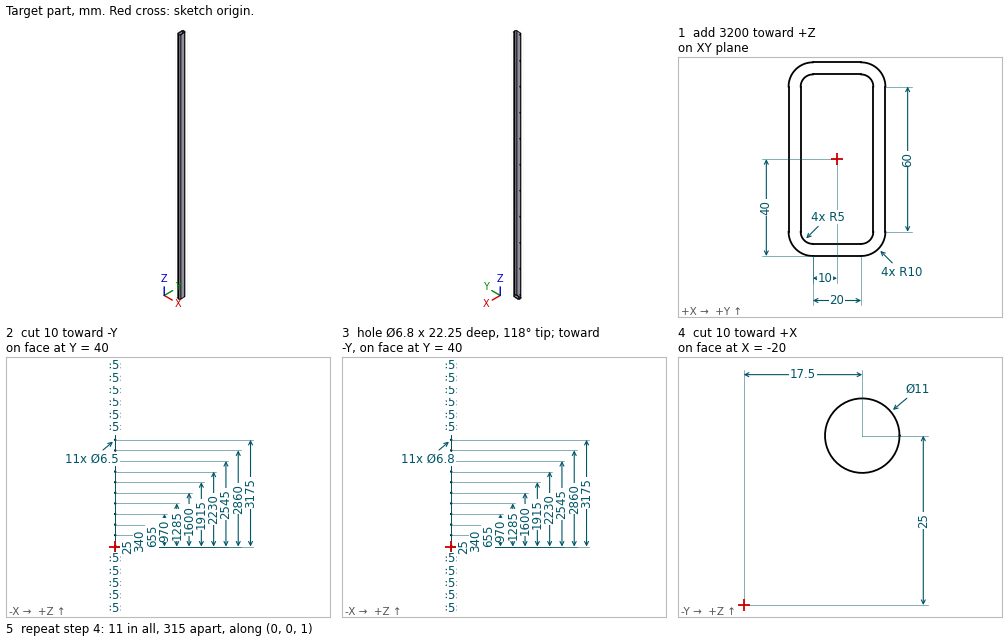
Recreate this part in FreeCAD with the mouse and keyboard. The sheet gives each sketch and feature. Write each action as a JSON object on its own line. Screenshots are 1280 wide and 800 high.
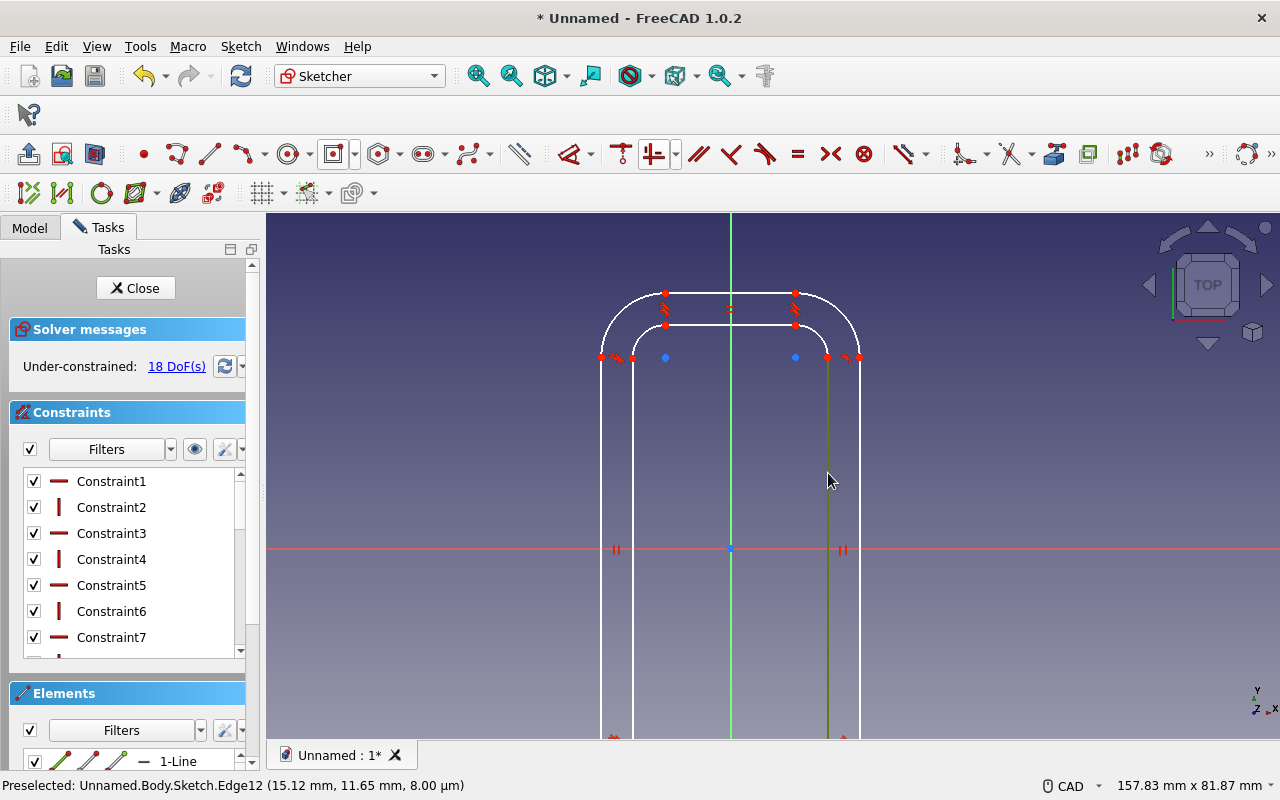
{"action": "left_click", "coordinate": [824, 343]}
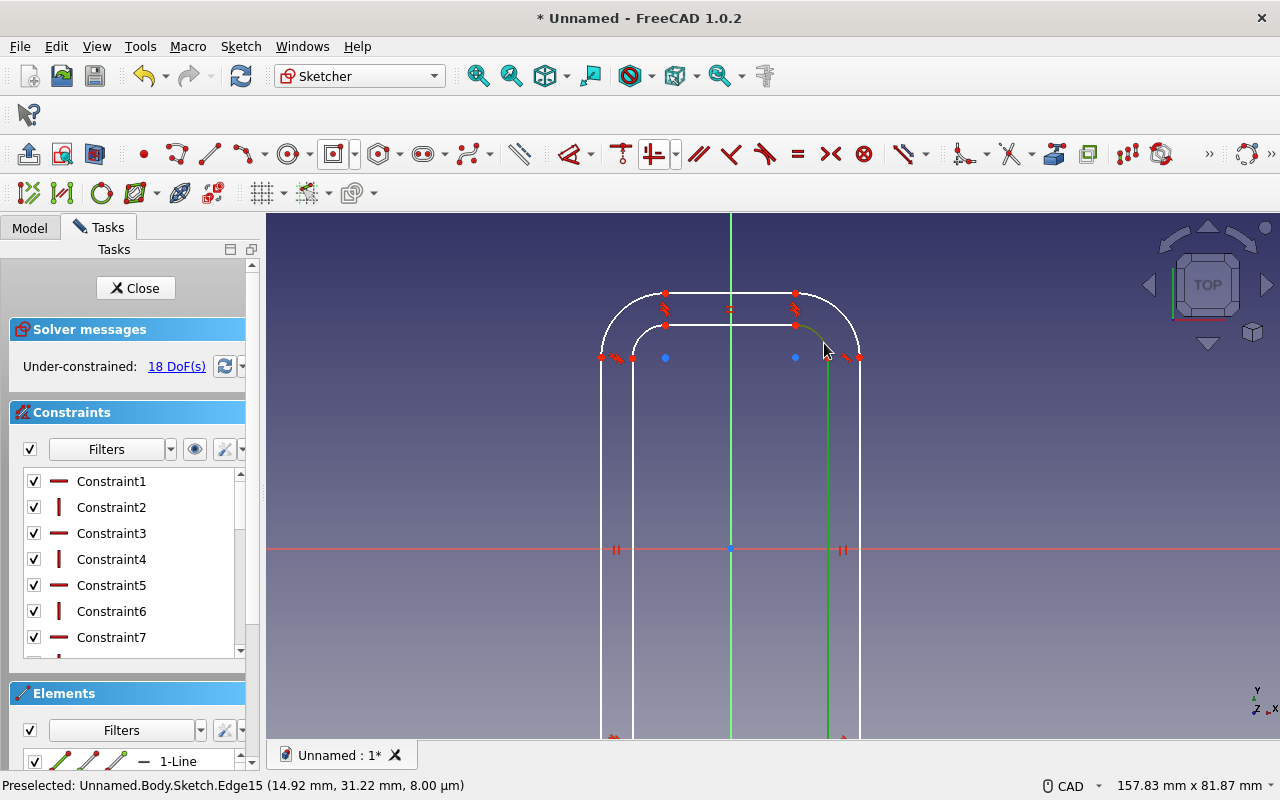
{"action": "left_click", "coordinate": [765, 154]}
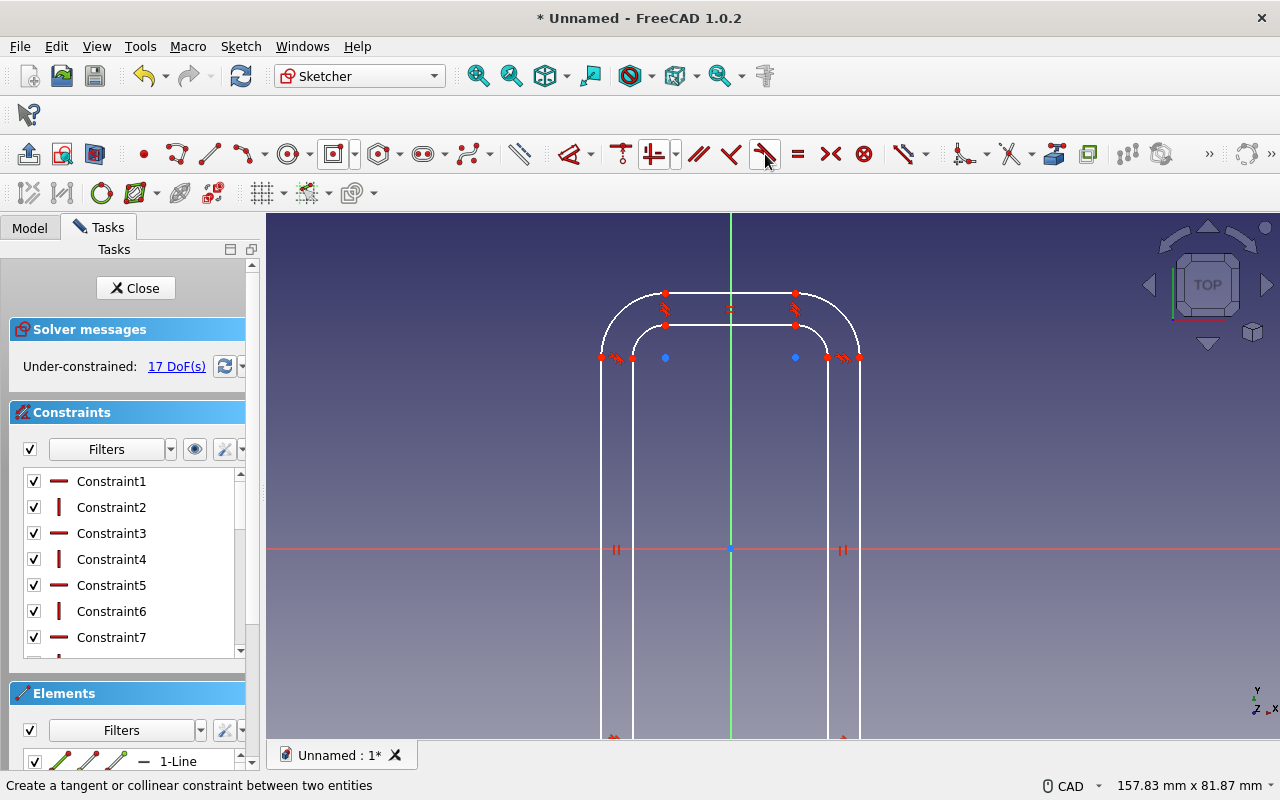
{"action": "left_click", "coordinate": [828, 473]}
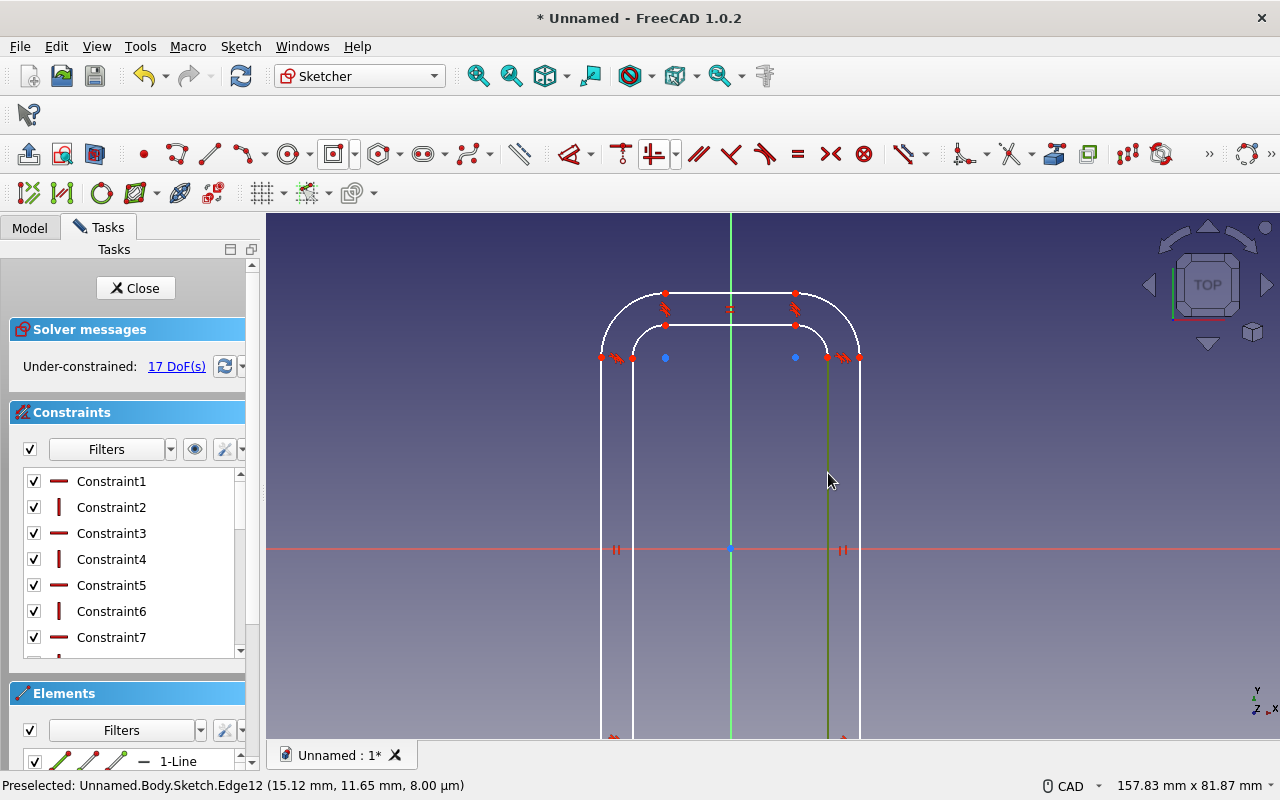
{"action": "scroll", "coordinate": [651, 328], "scroll_direction": "down", "scroll_amount": 2}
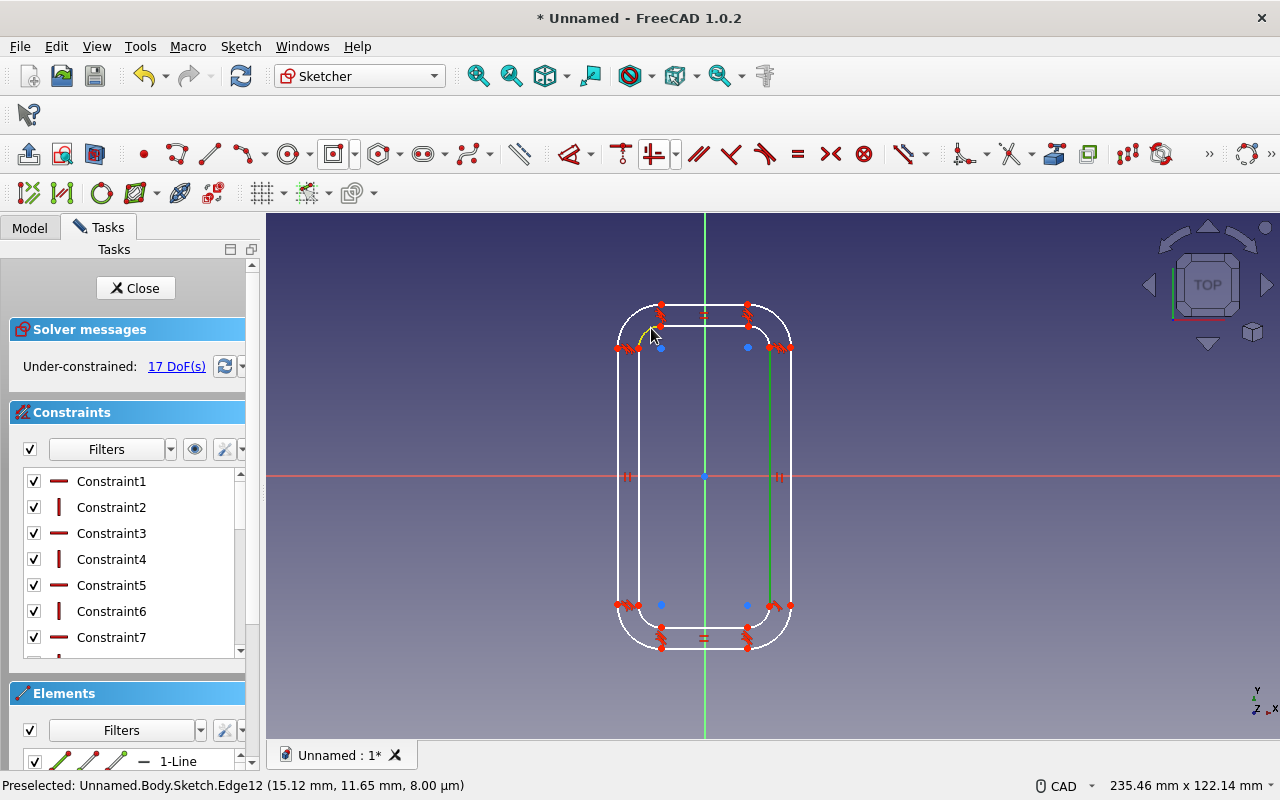
{"action": "scroll", "coordinate": [757, 625], "scroll_direction": "up", "scroll_amount": 2}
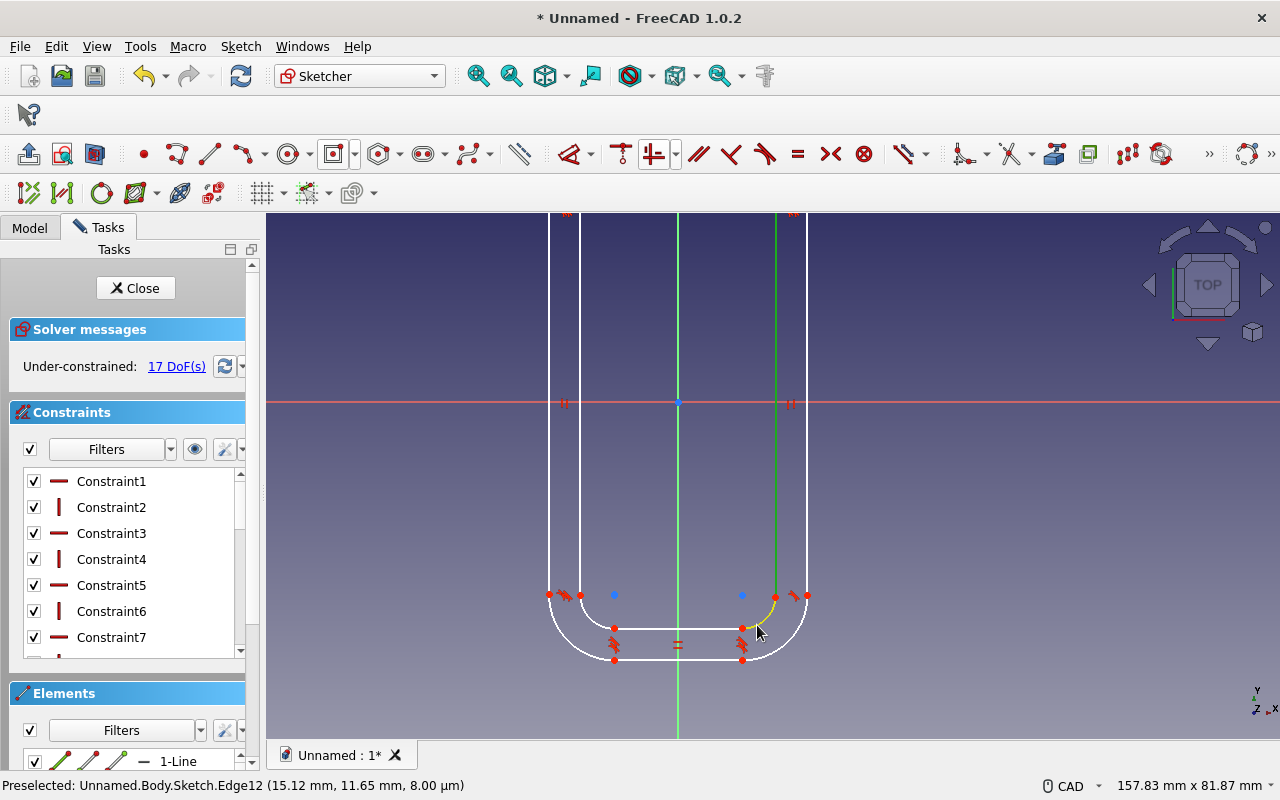
{"action": "left_click", "coordinate": [757, 625]}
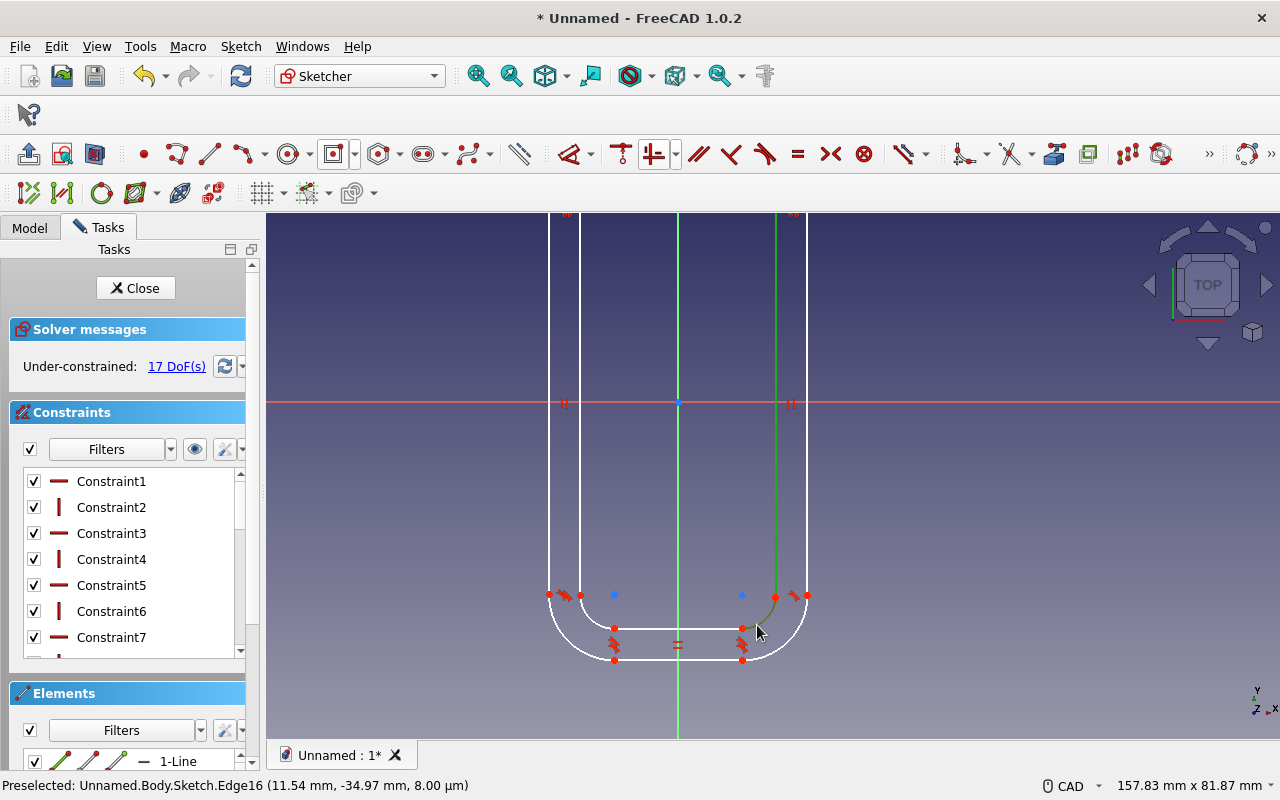
{"action": "left_click", "coordinate": [765, 154]}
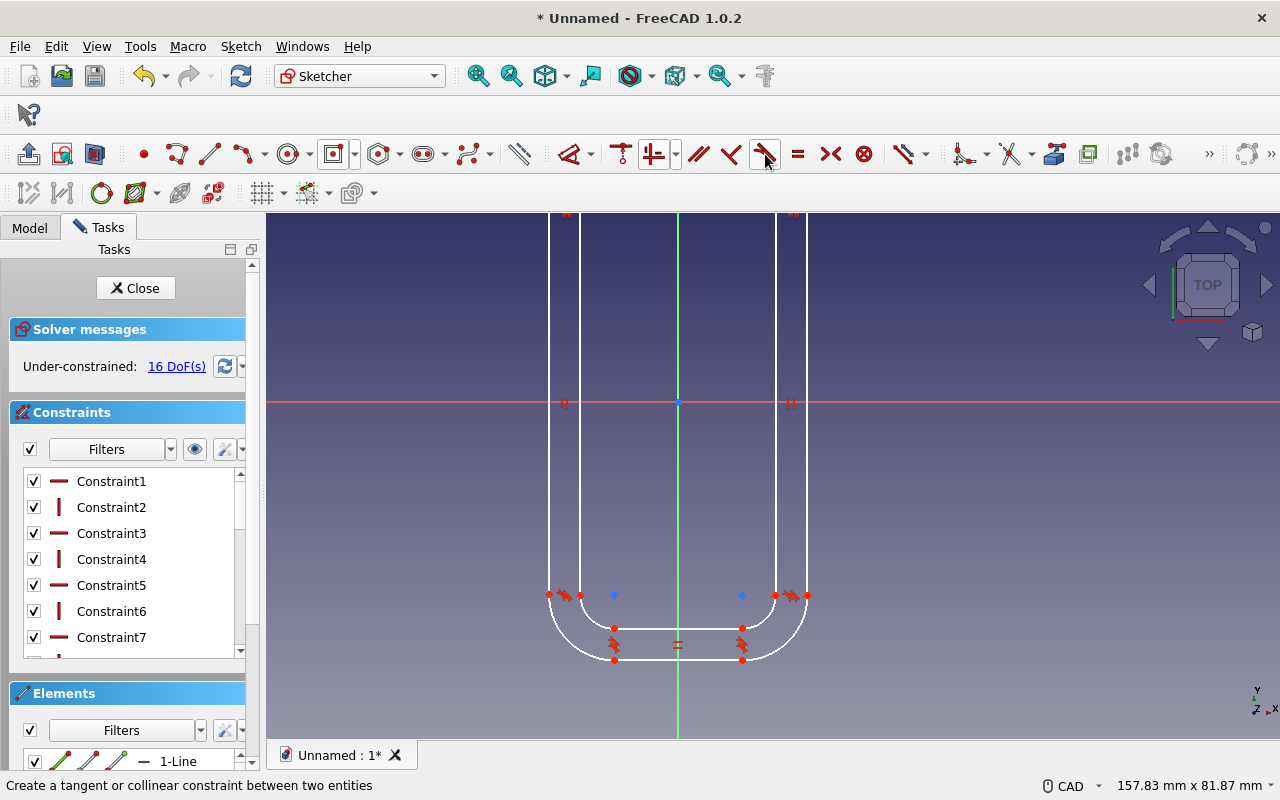
{"action": "left_click", "coordinate": [556, 624]}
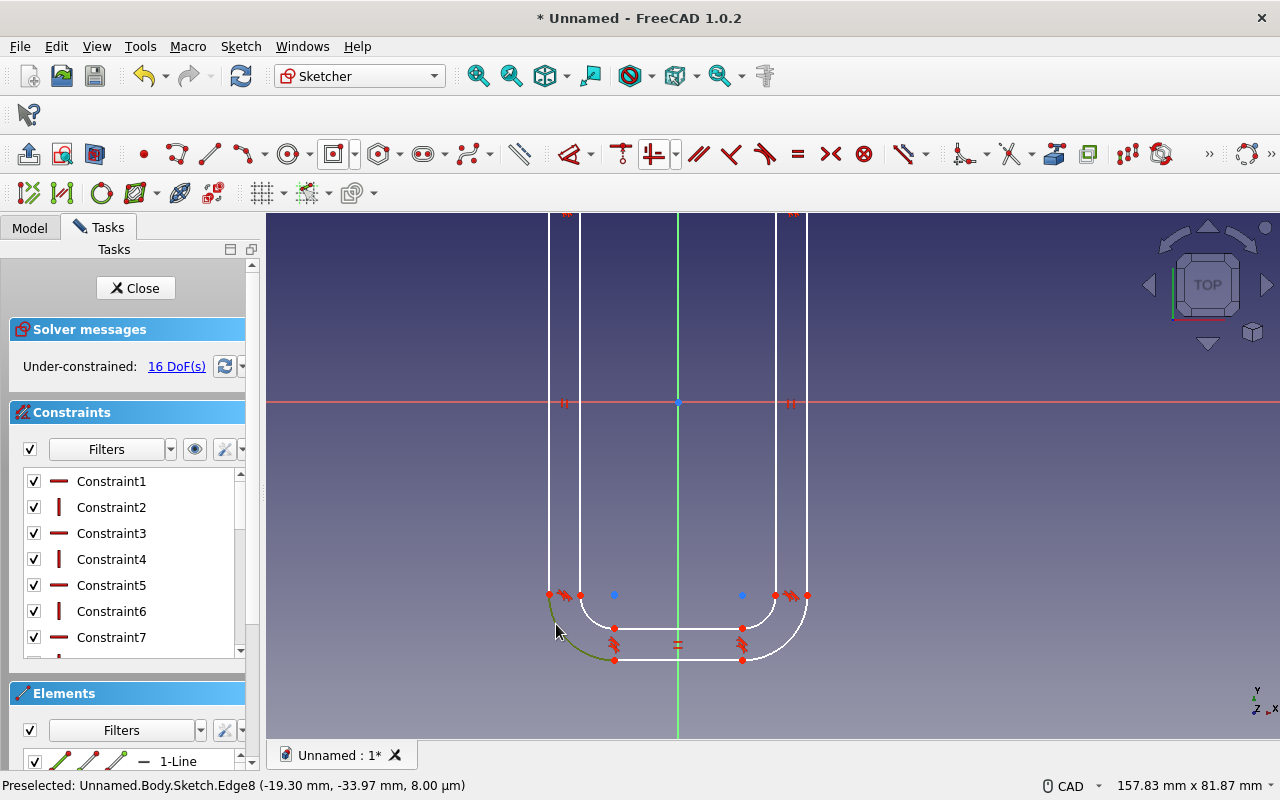
{"action": "left_click", "coordinate": [584, 610]}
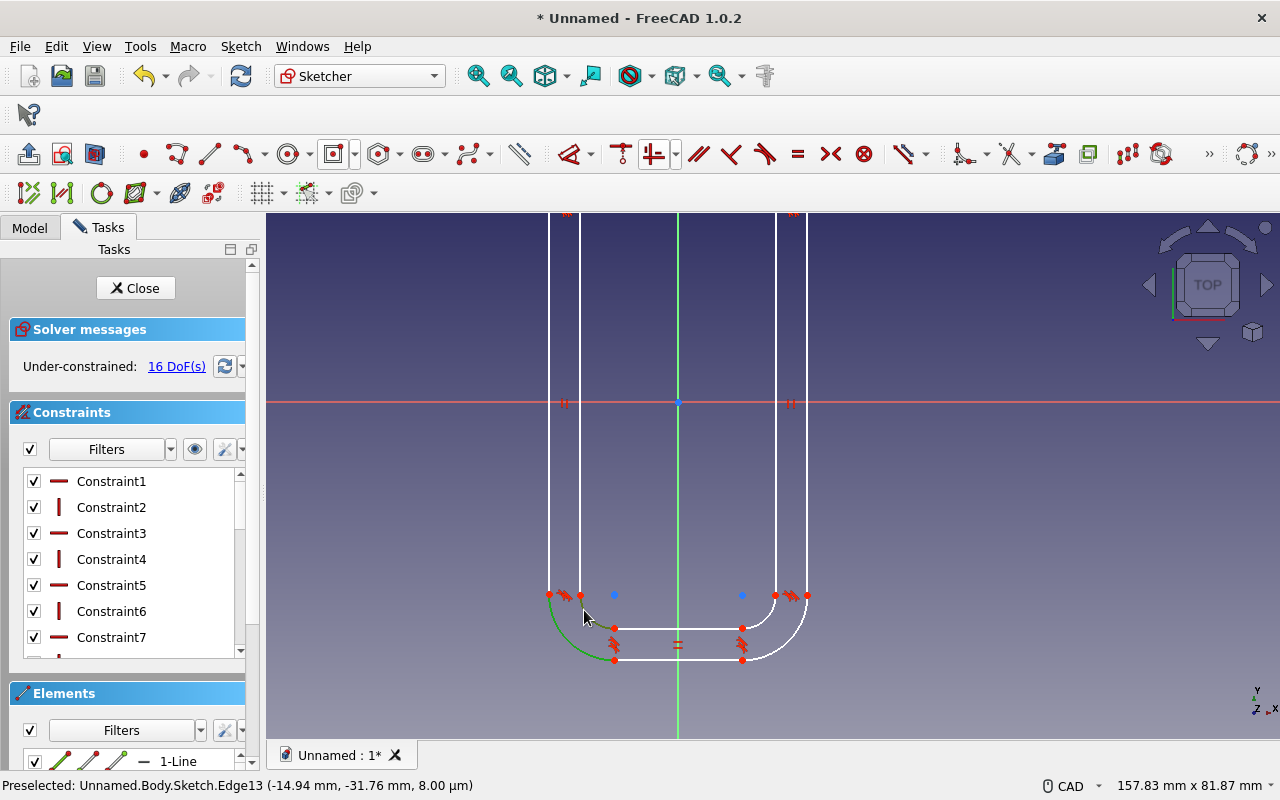
{"action": "key", "text": "c"}